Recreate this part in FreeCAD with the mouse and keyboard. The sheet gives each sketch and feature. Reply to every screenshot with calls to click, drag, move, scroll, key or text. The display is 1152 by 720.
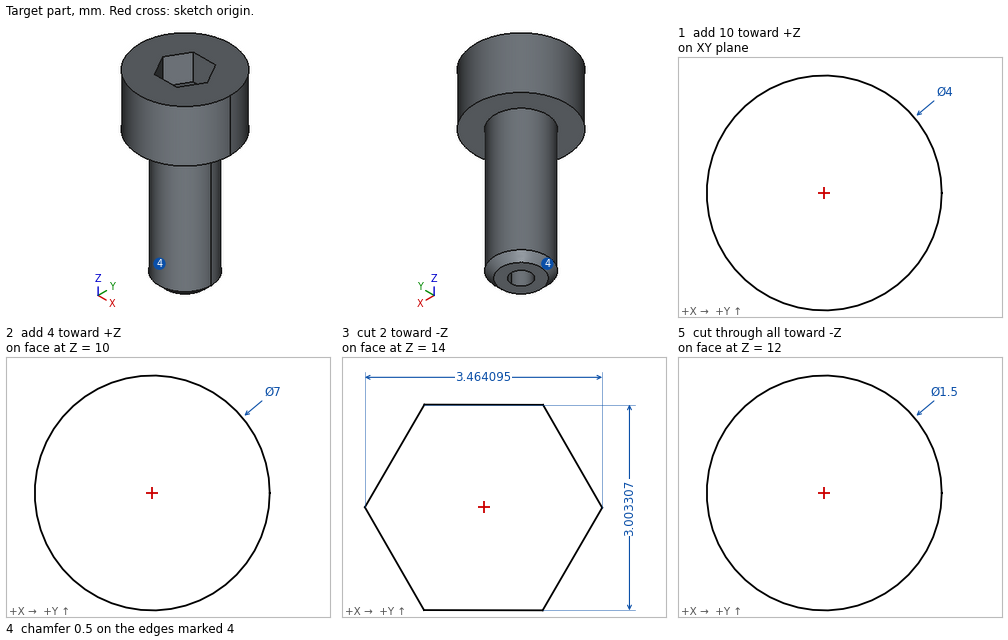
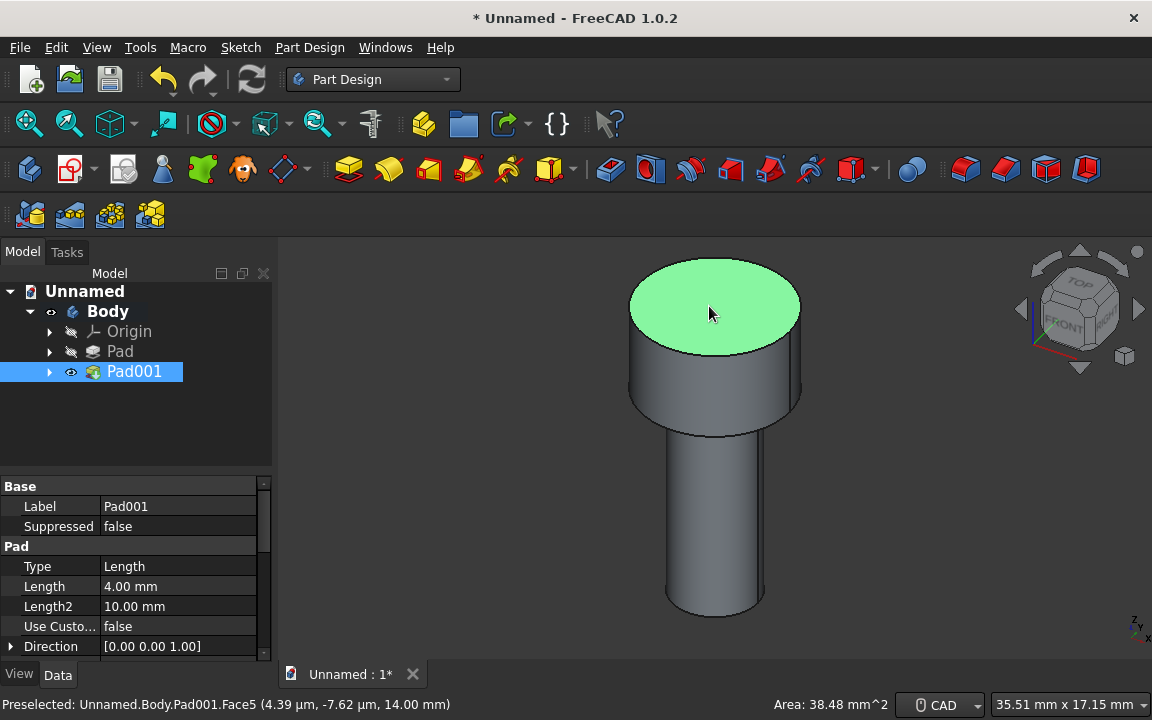
click(70, 170)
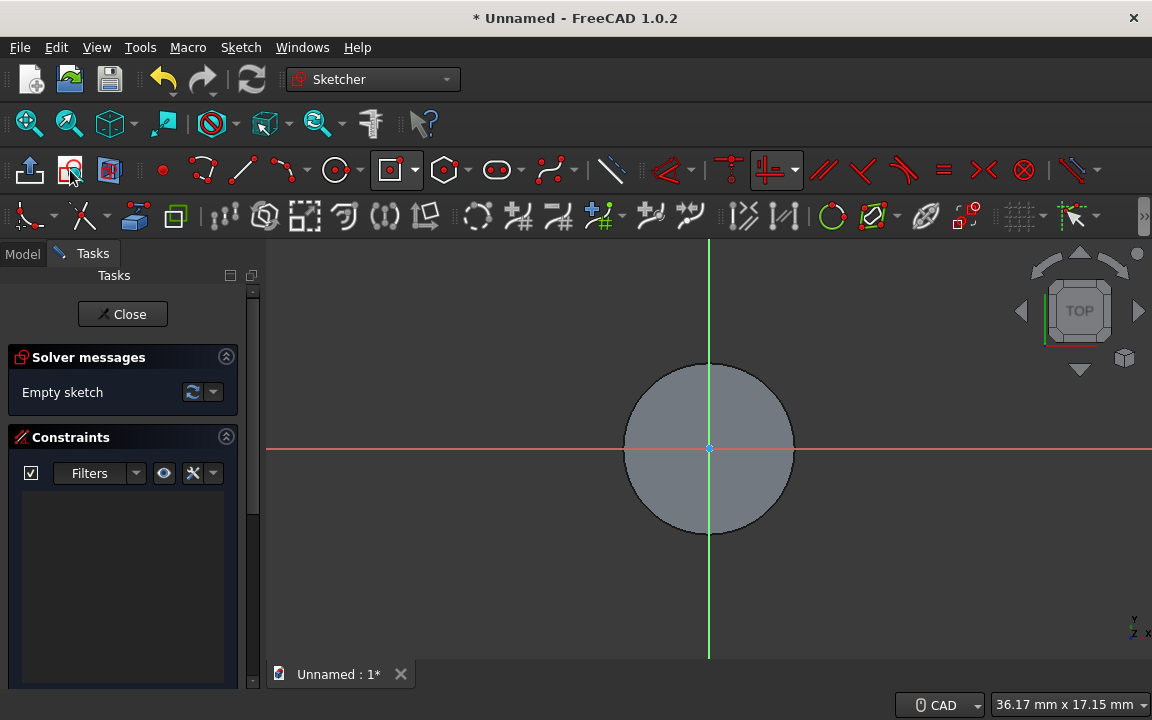
scroll(739, 449, up, 6)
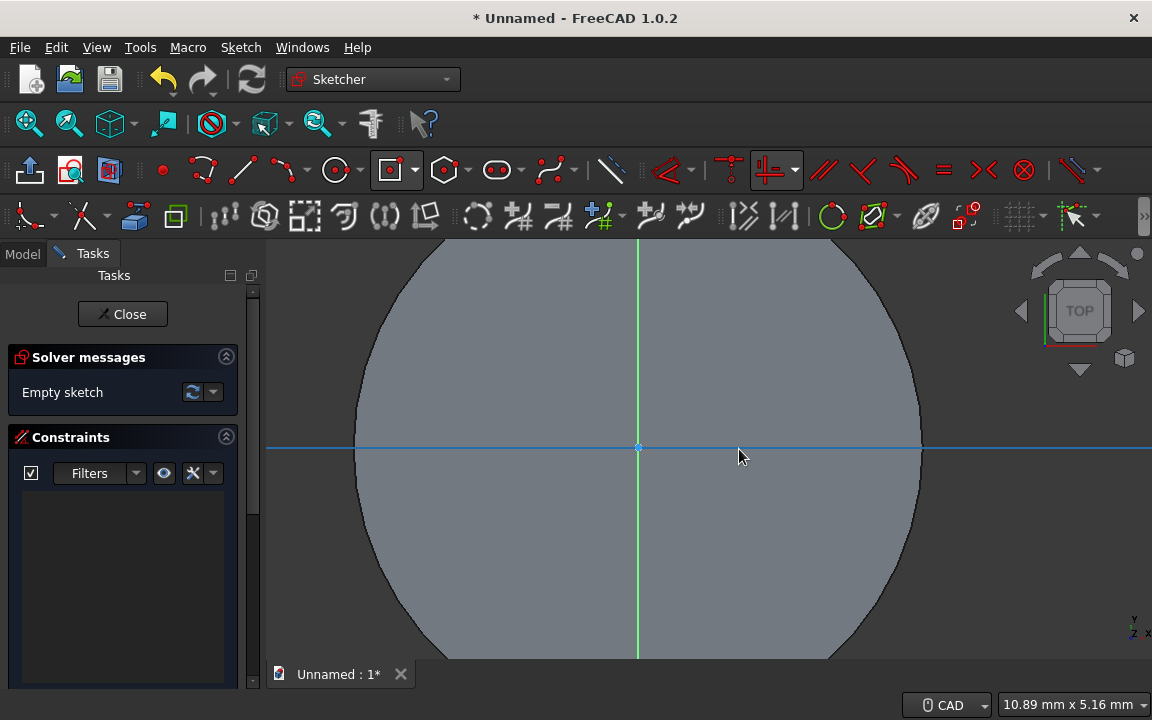
click(444, 170)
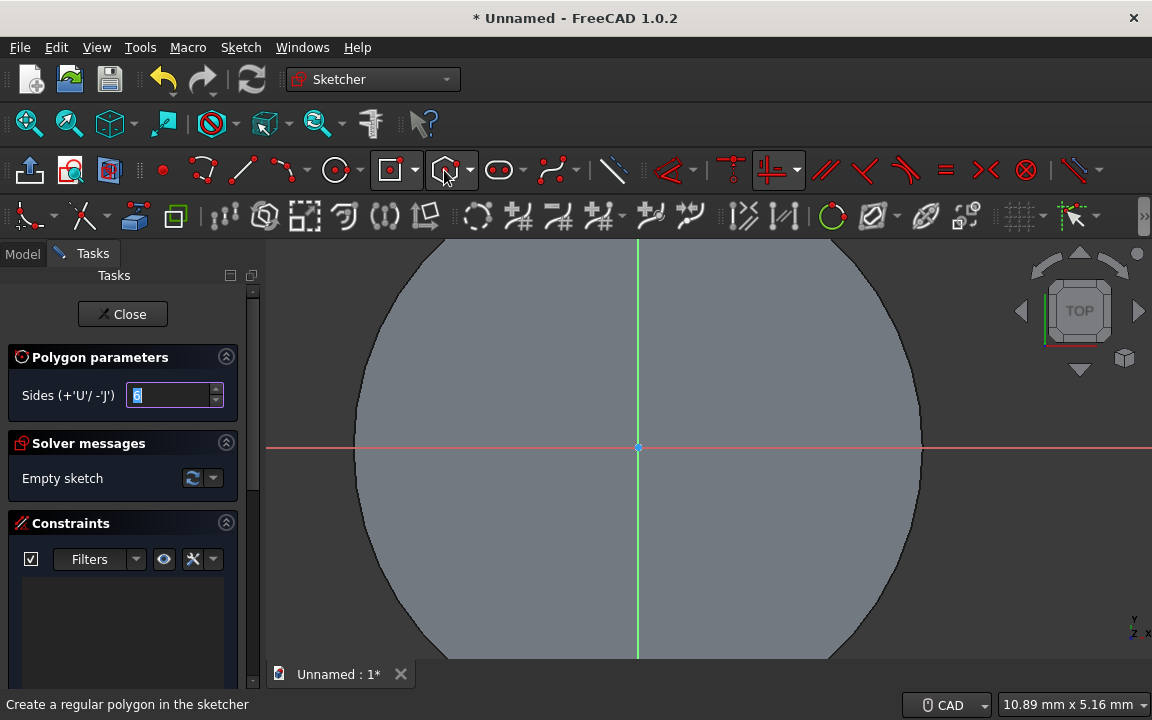
click(638, 448)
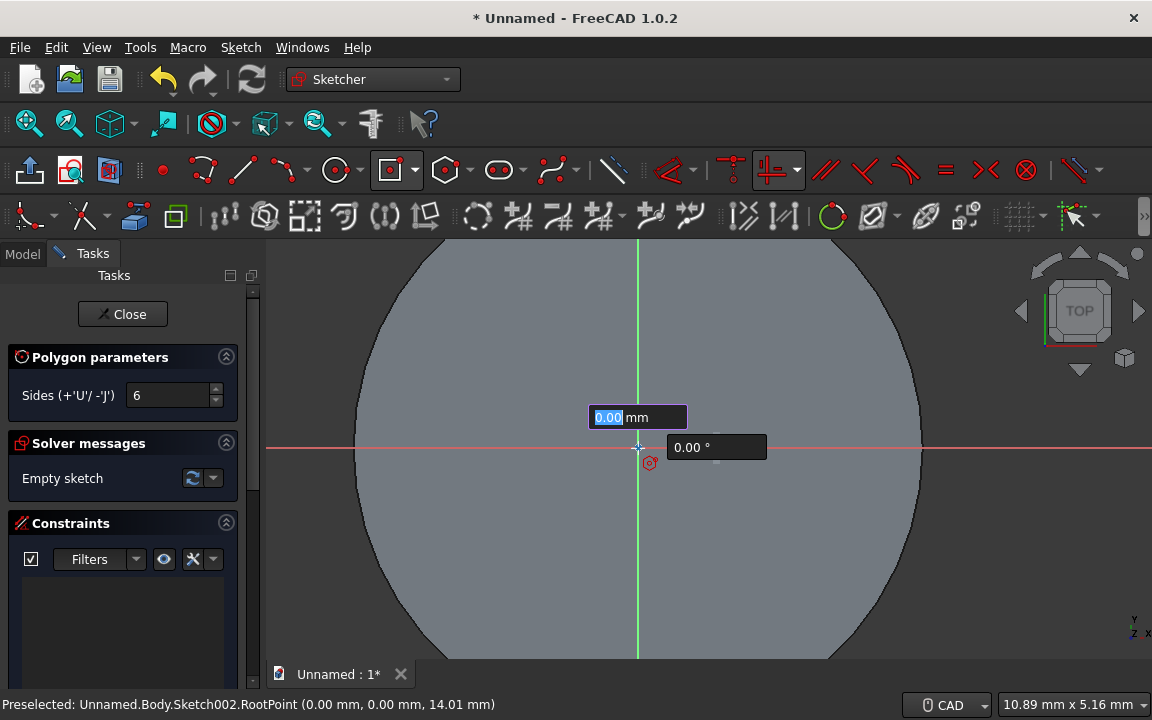
click(567, 570)
right_click(567, 570)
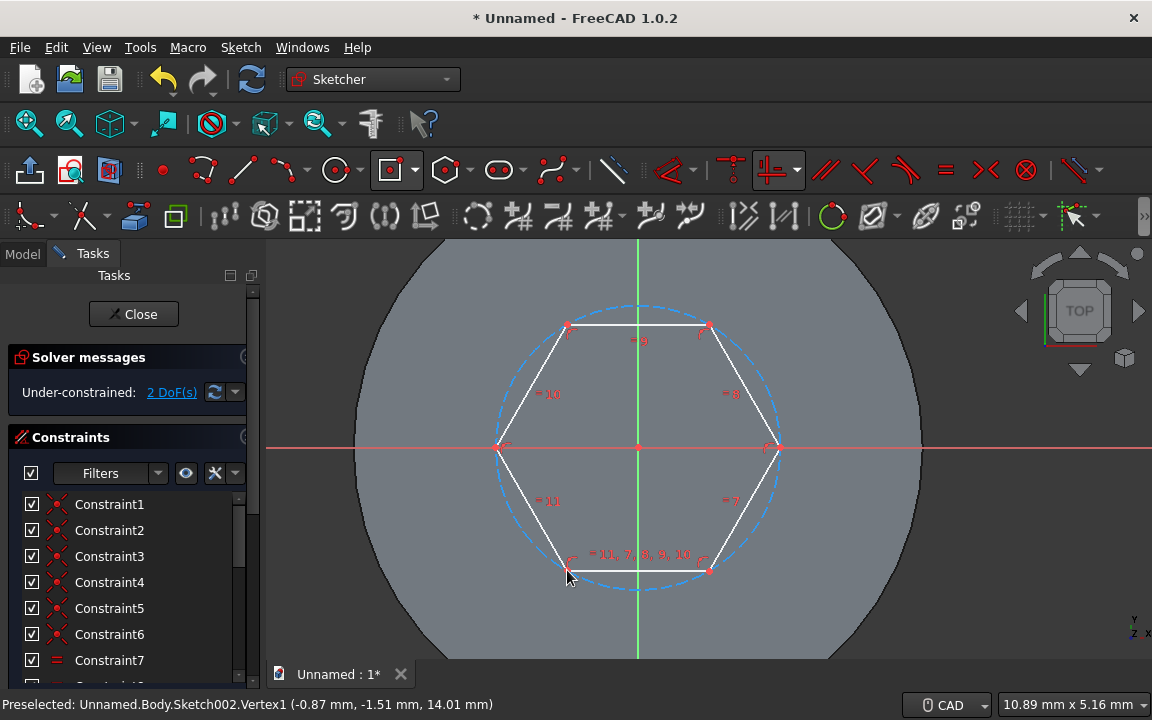
click(668, 170)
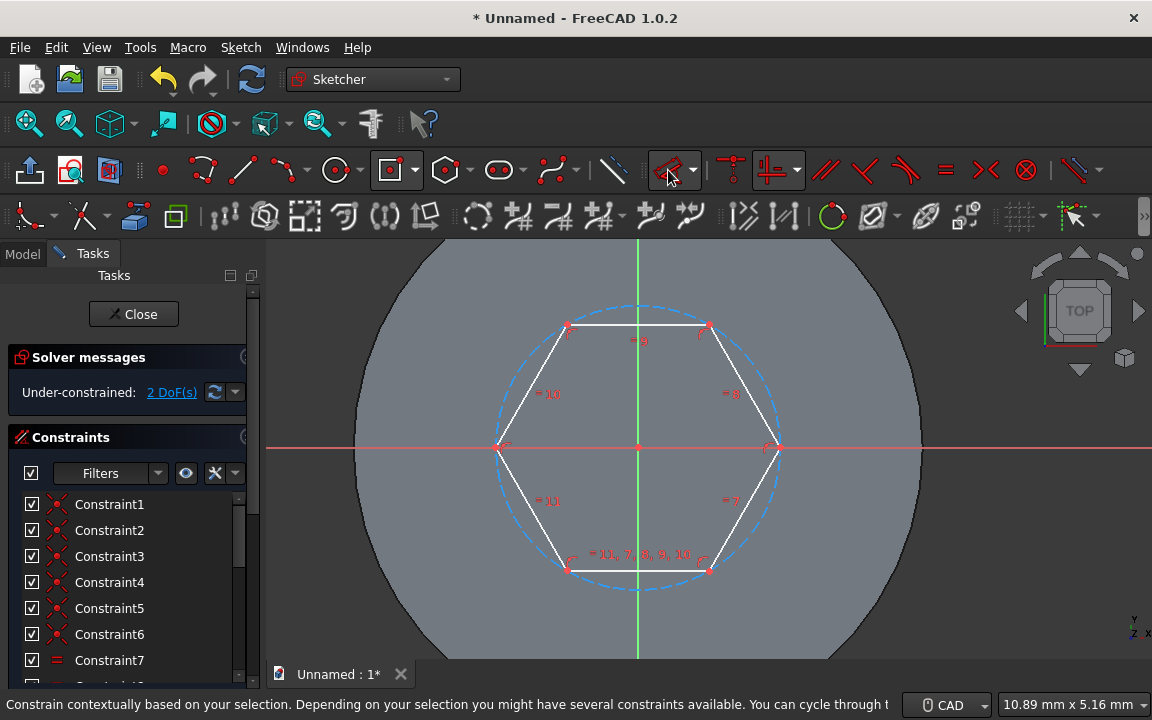
click(496, 448)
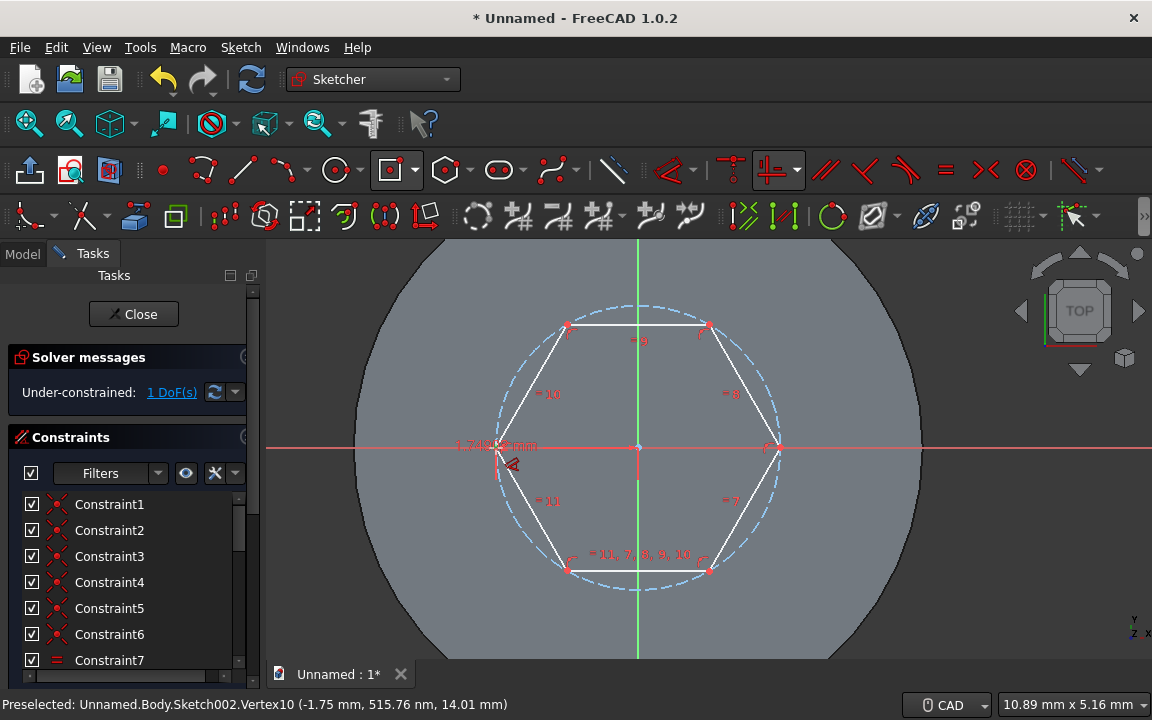
click(780, 448)
click(573, 414)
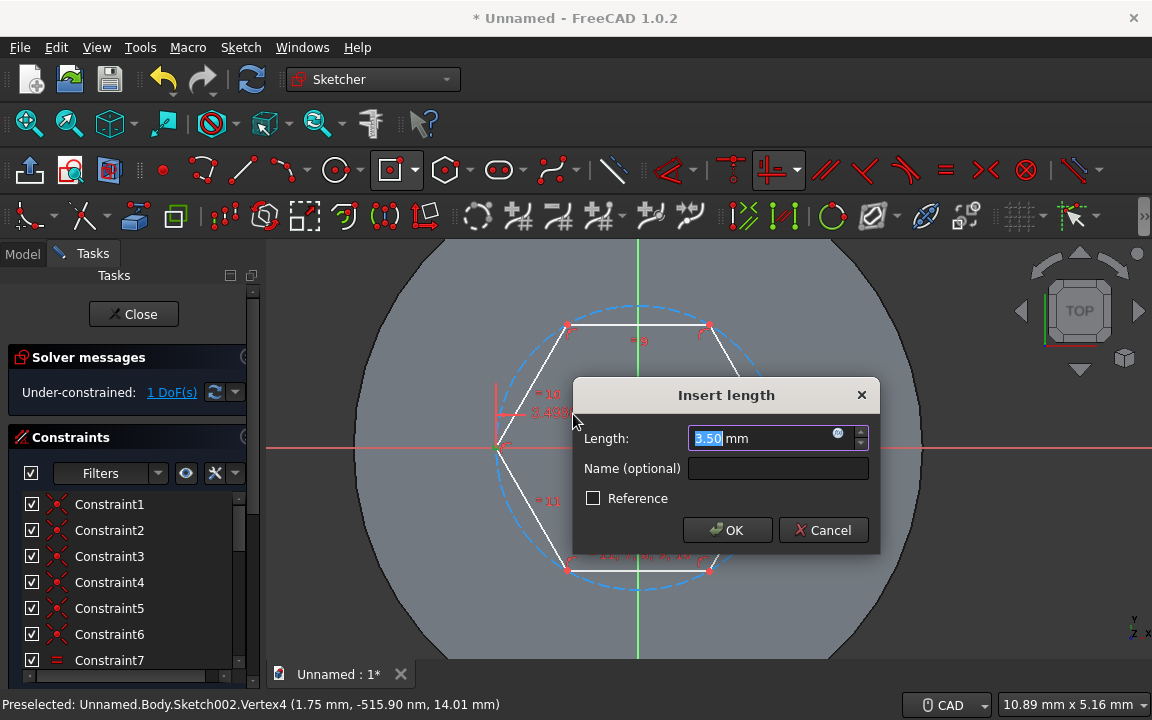
text(3.464095)
key(Return)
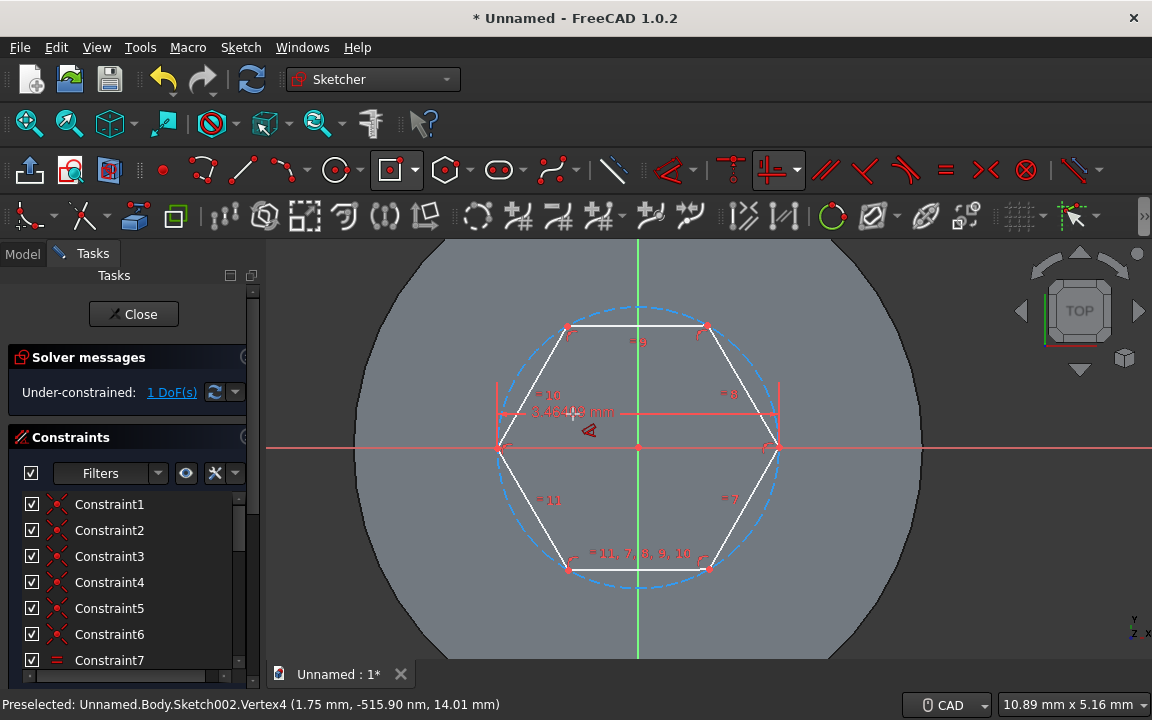
click(709, 569)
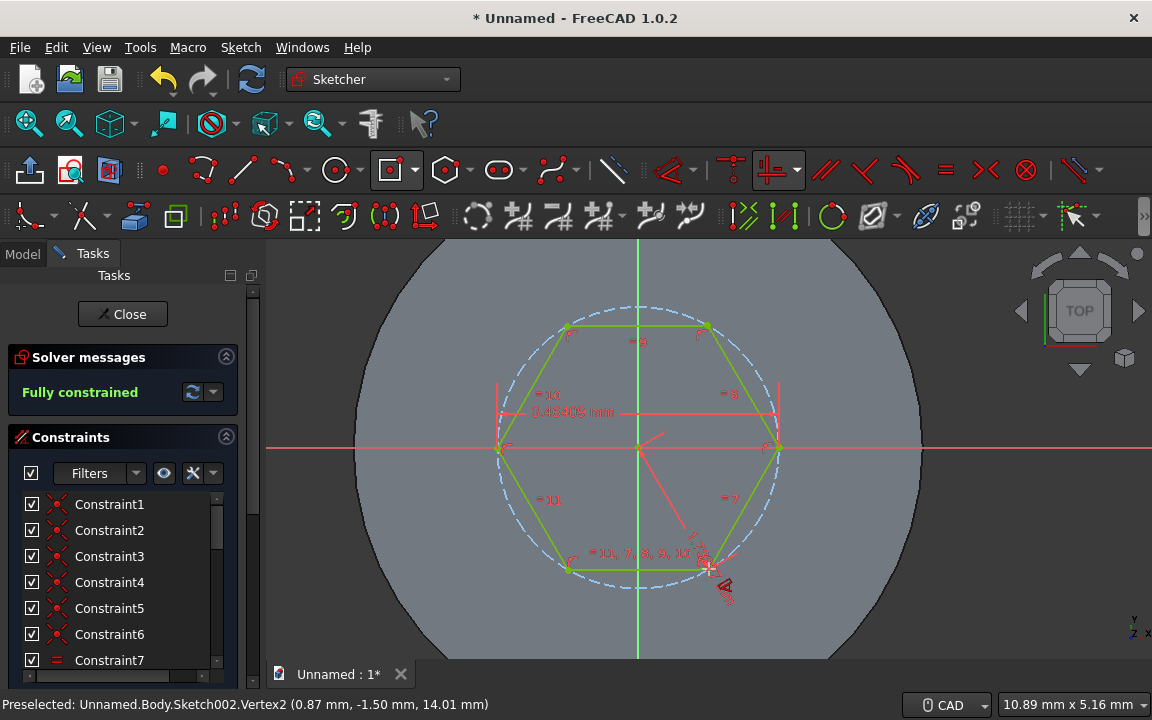
click(567, 326)
click(767, 363)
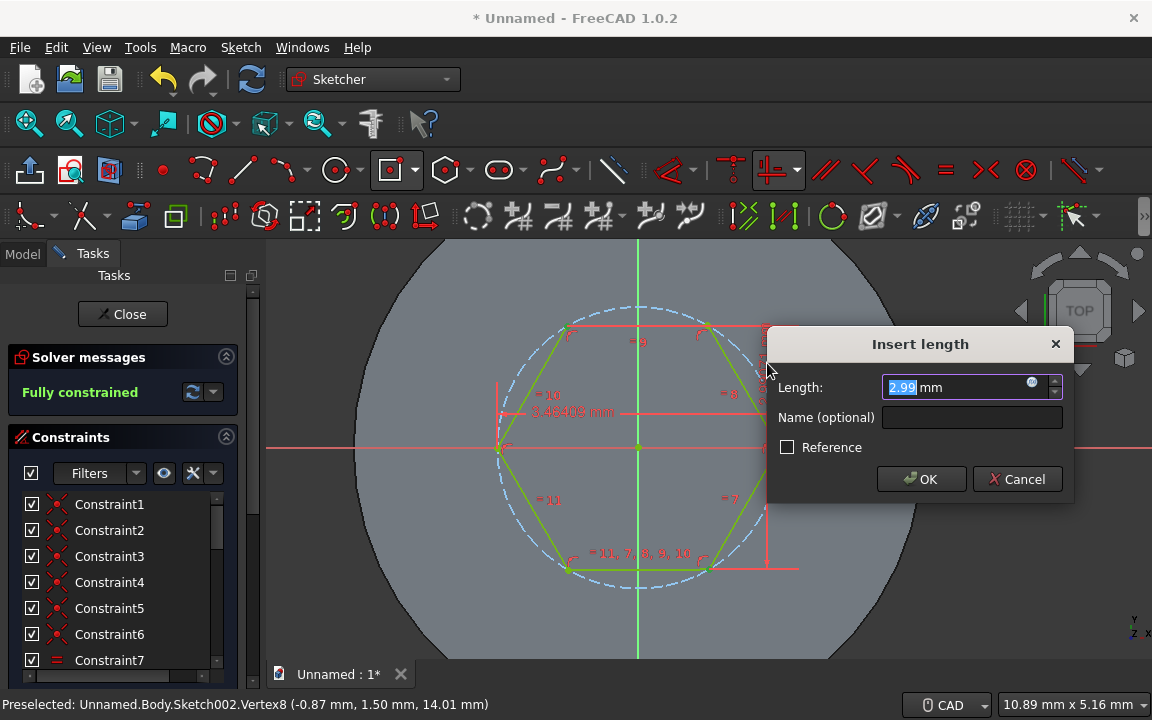
text(3.003307)
key(Return)
key(Escape)